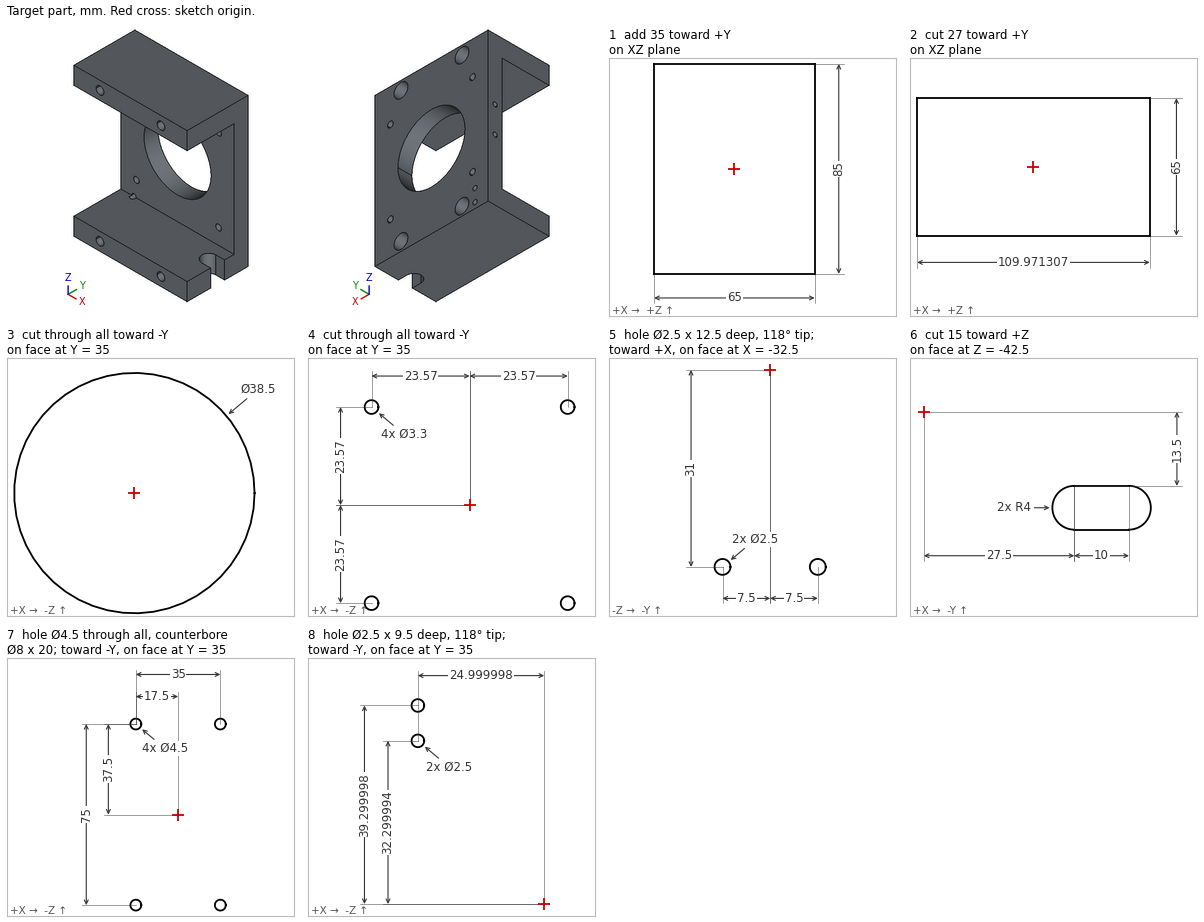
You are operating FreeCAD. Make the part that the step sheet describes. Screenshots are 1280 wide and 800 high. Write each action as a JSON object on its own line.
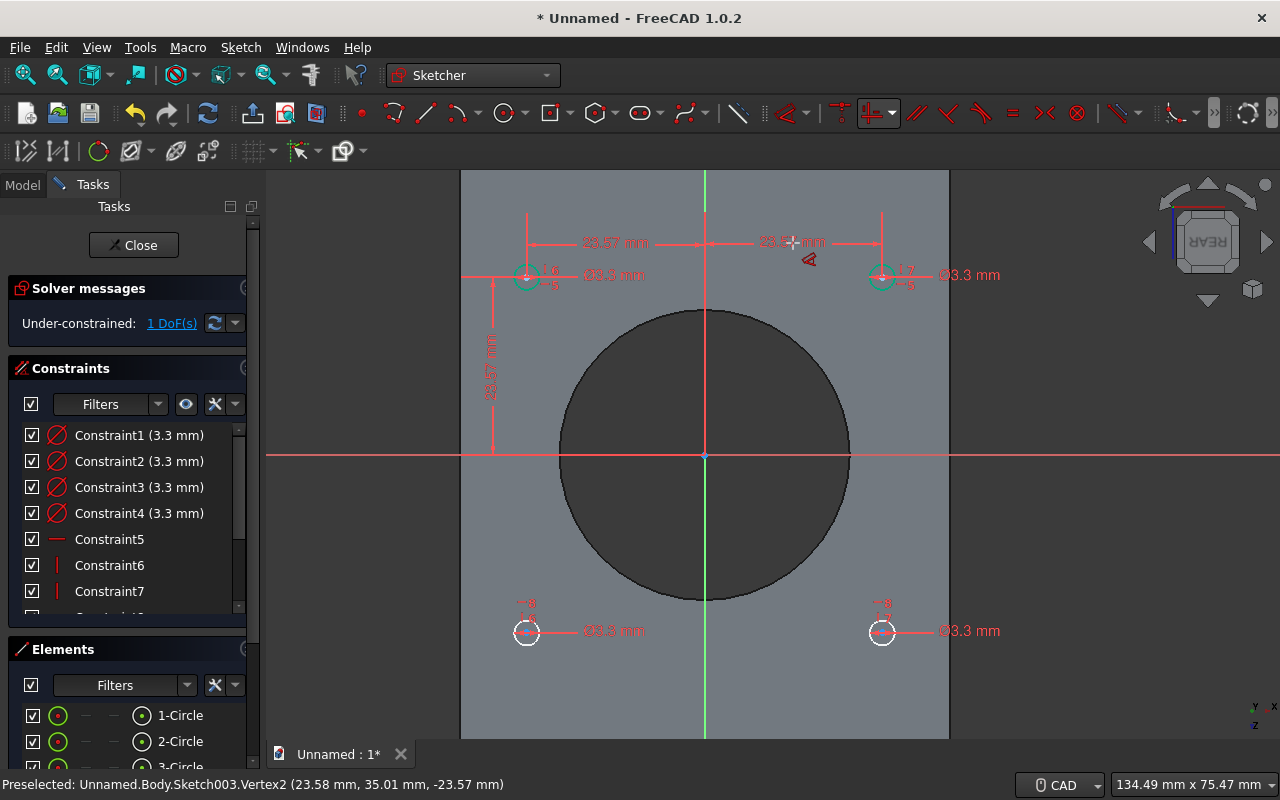
{"action": "left_click", "coordinate": [527, 633]}
{"action": "left_click", "coordinate": [493, 544]}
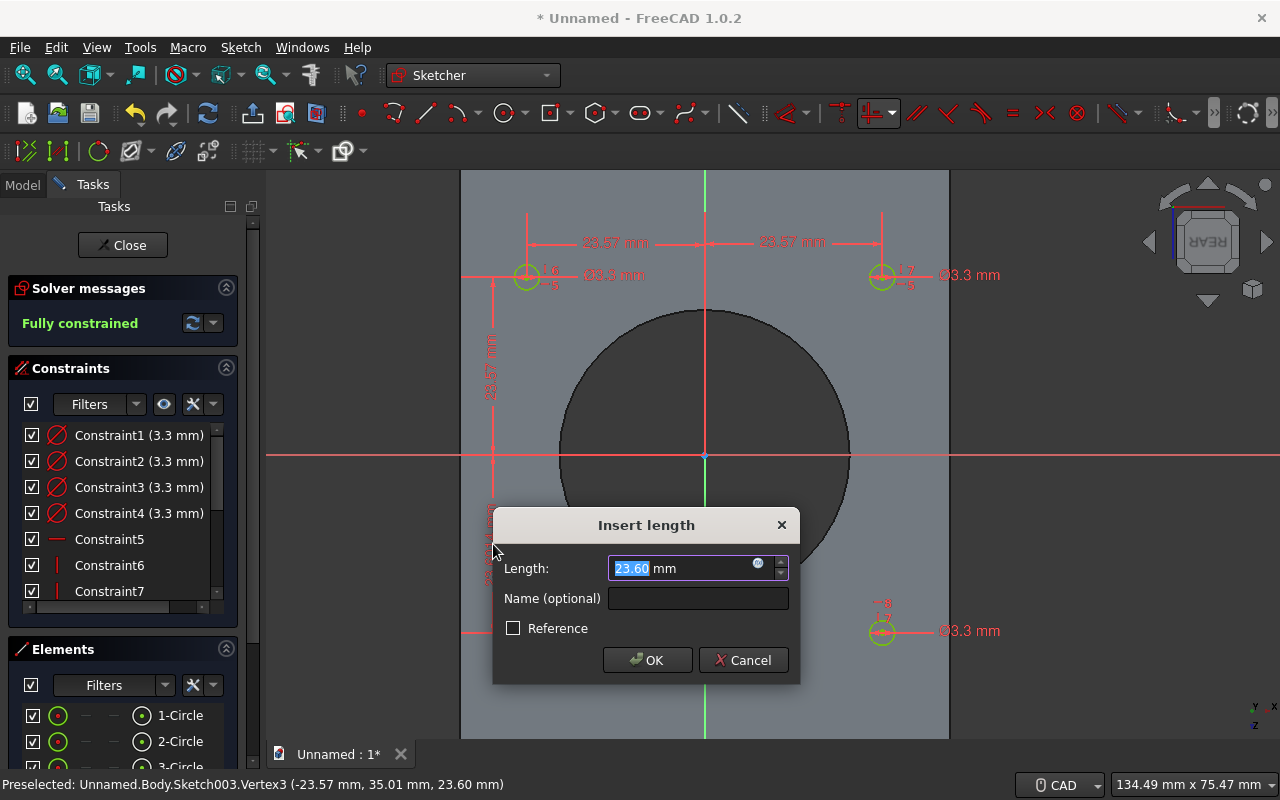
{"action": "type", "text": "23.57"}
{"action": "key", "text": "Return"}
{"action": "key", "text": "Escape"}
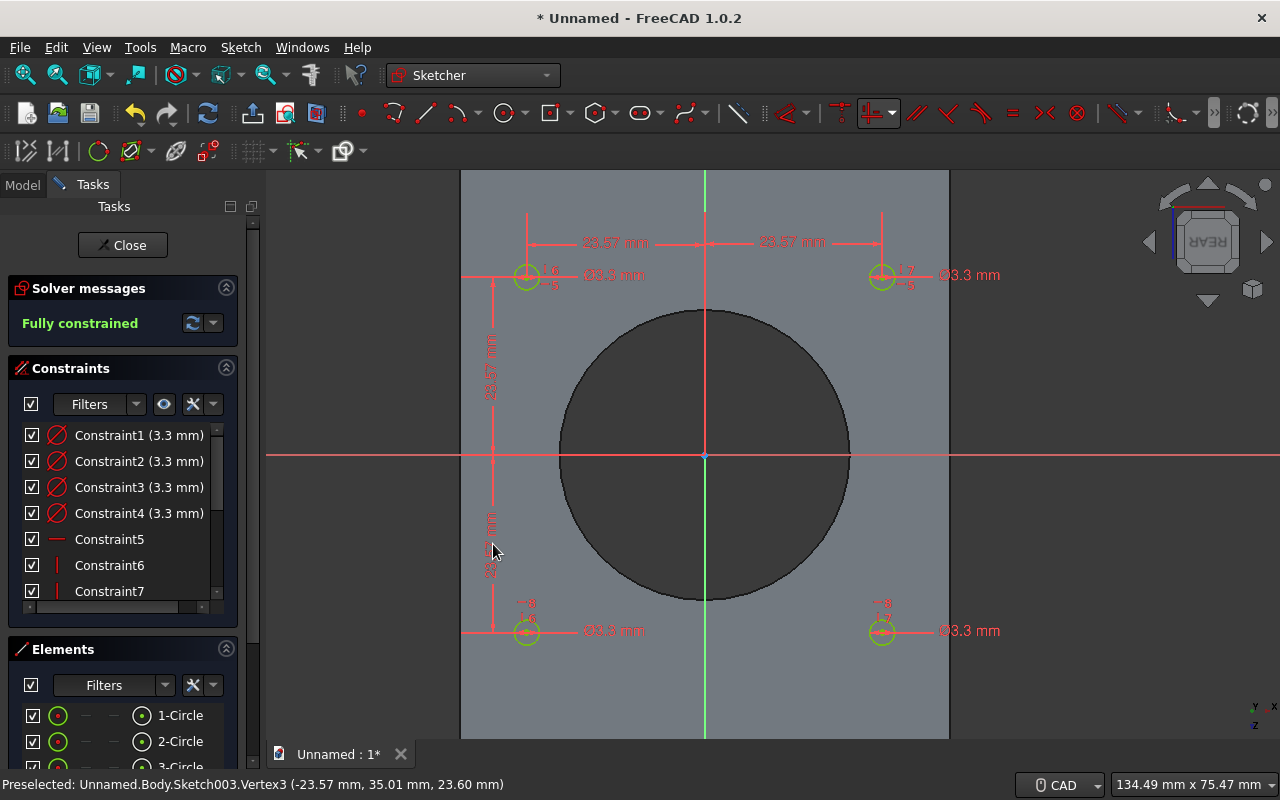
{"action": "left_click", "coordinate": [123, 245]}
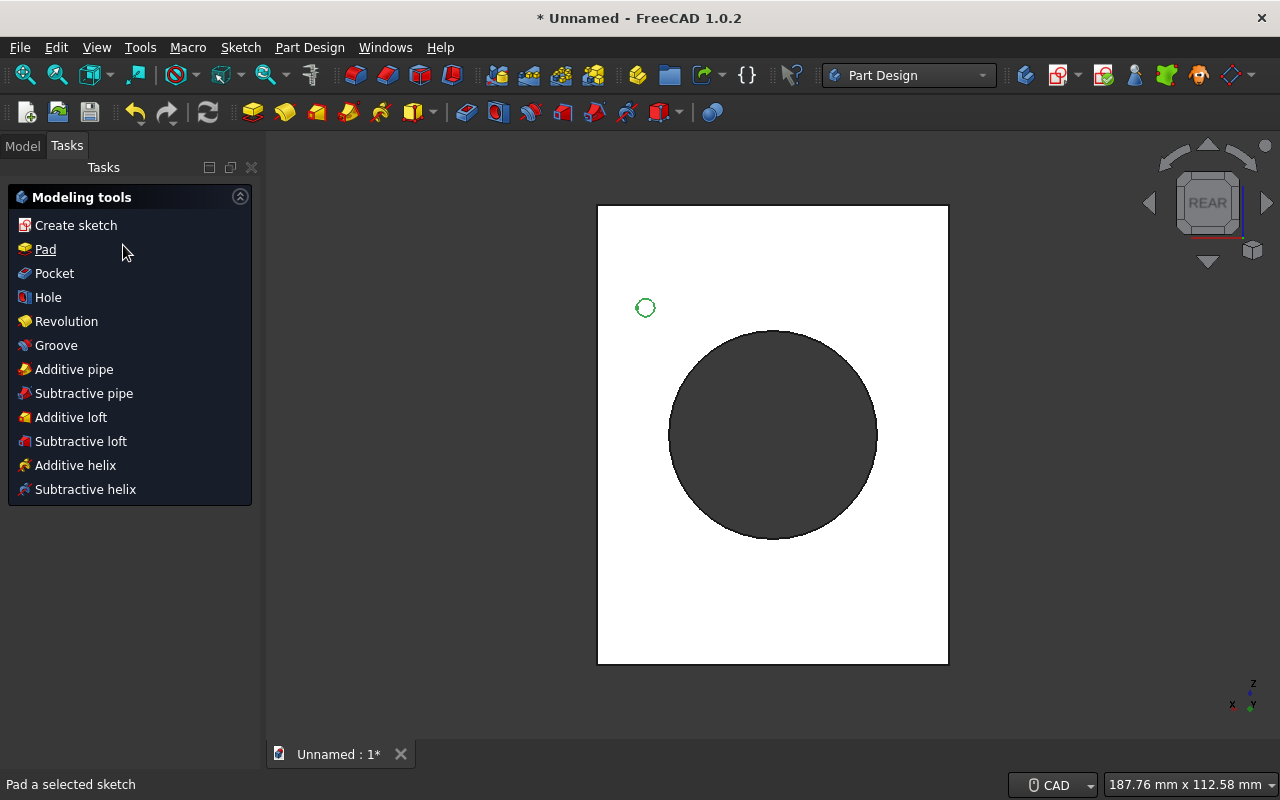
{"action": "left_click", "coordinate": [468, 112]}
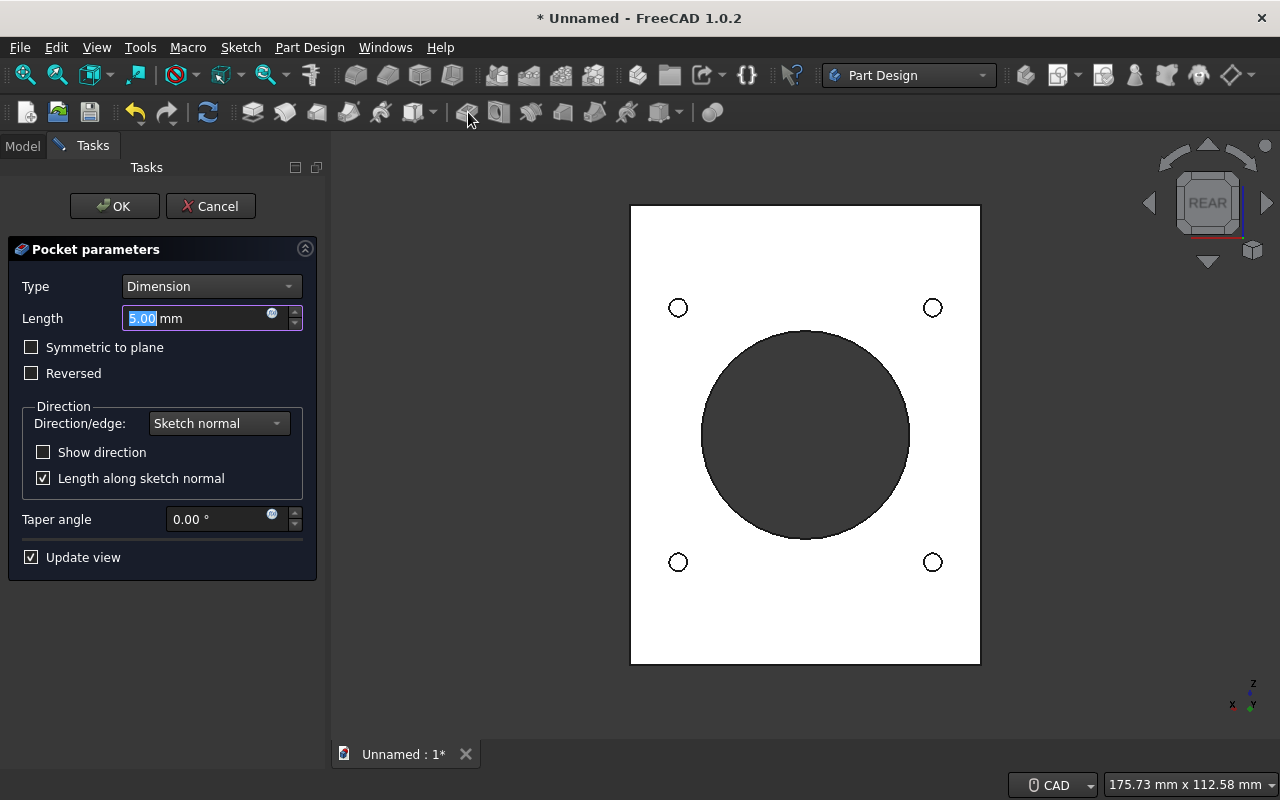
{"action": "left_click", "coordinate": [212, 286]}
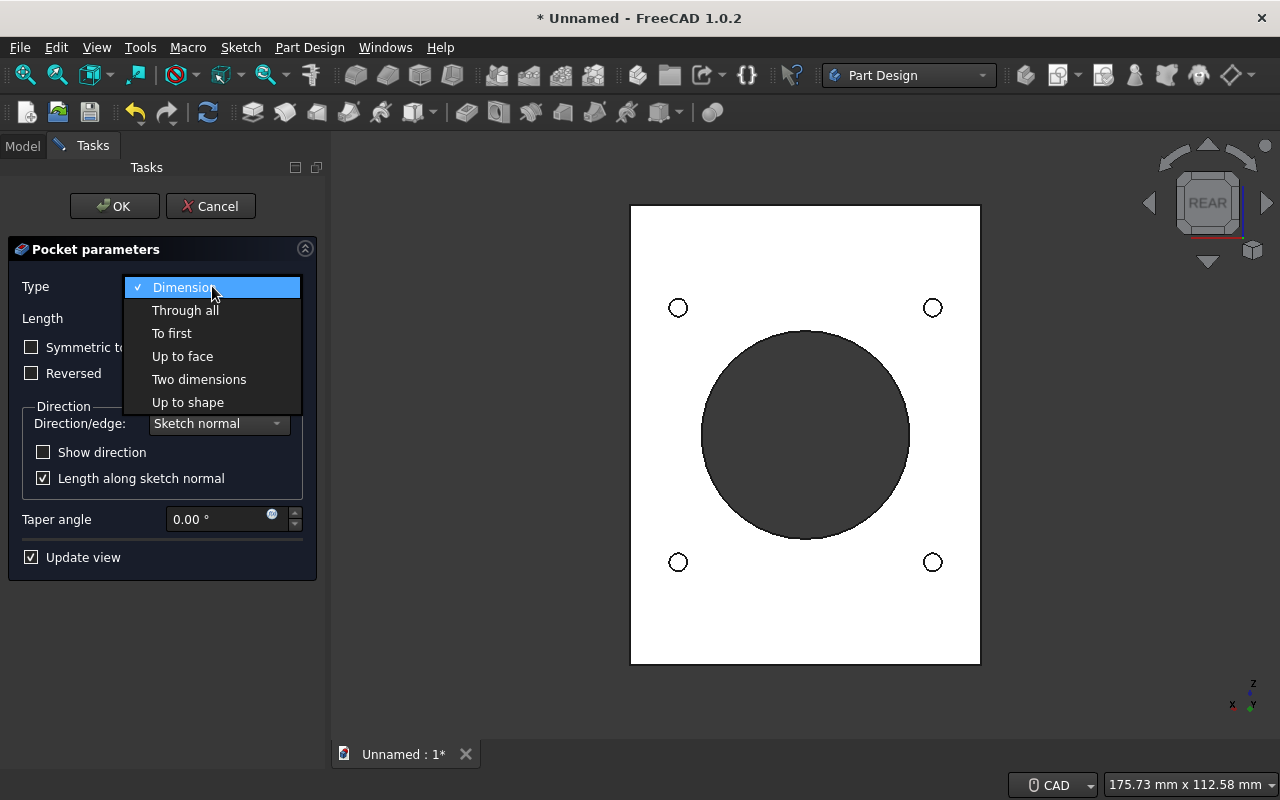
{"action": "left_click", "coordinate": [212, 310]}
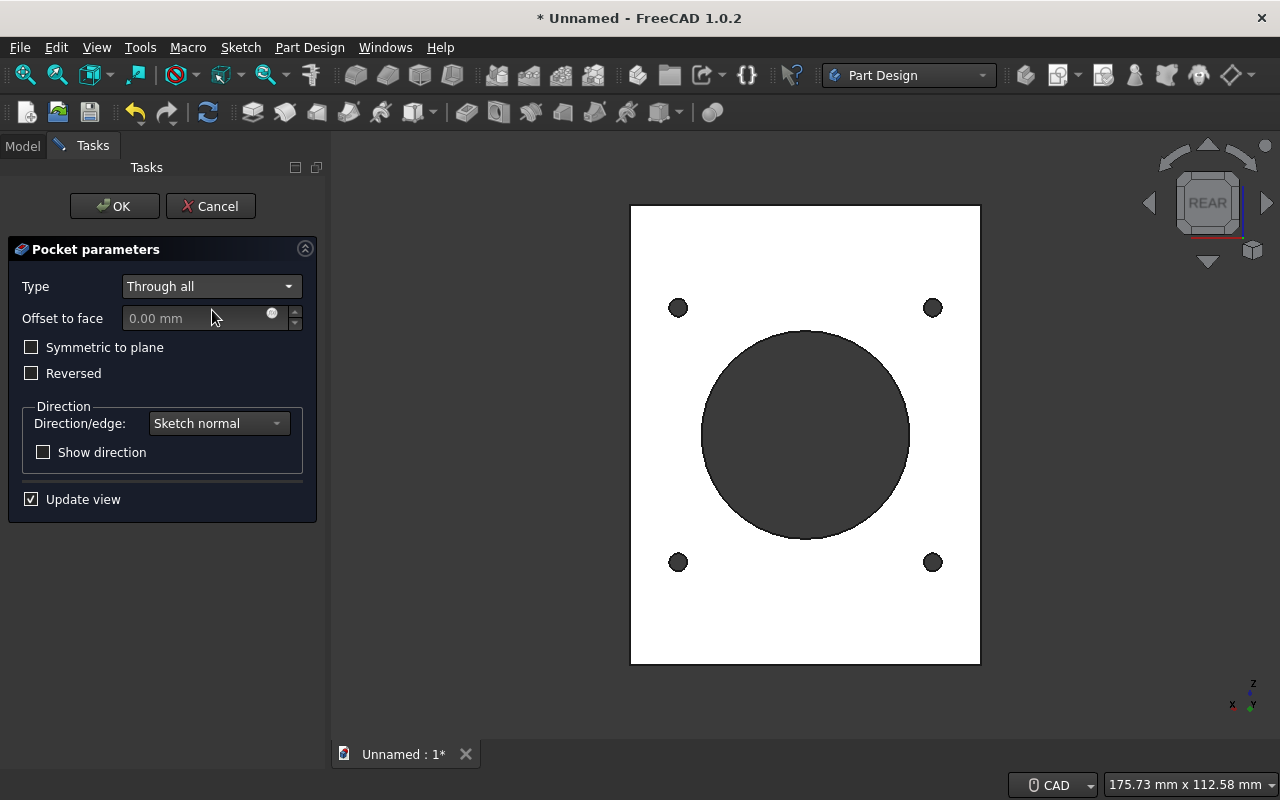
{"action": "left_click", "coordinate": [115, 206]}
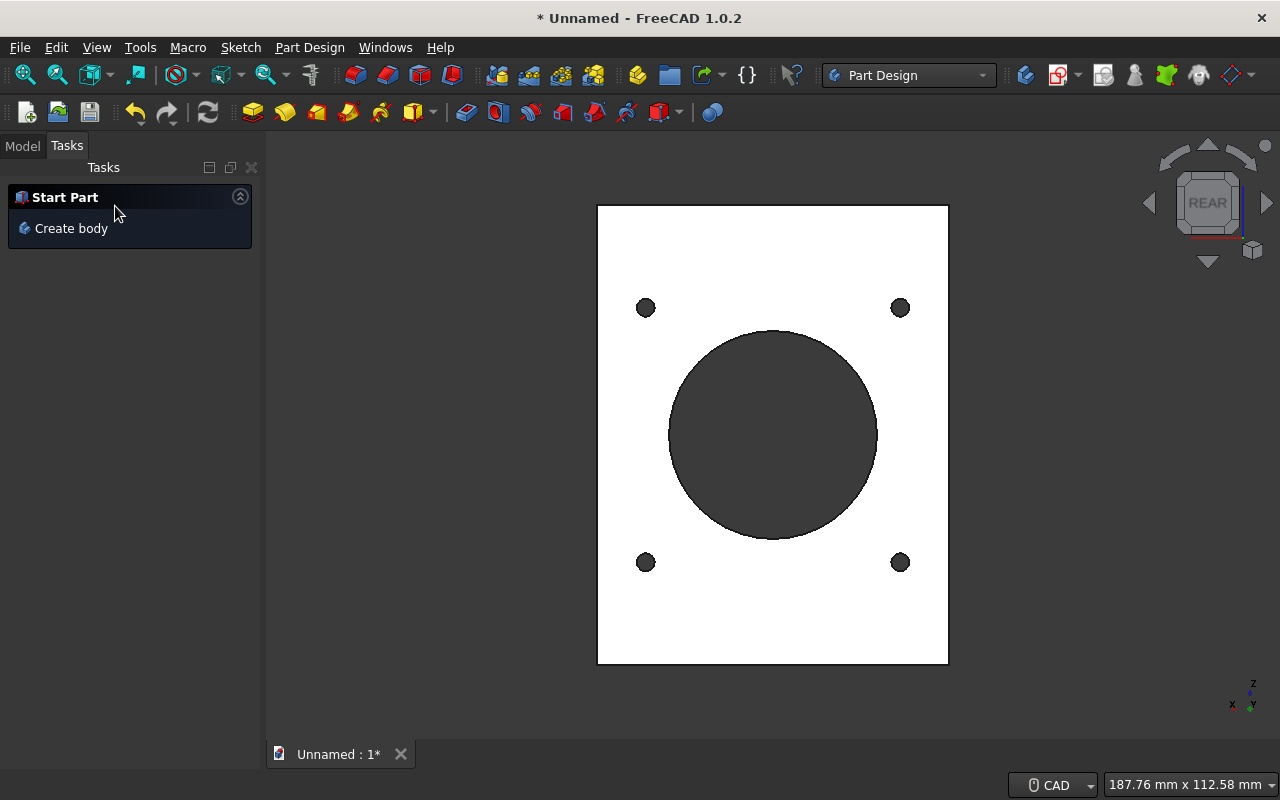
{"action": "key", "text": "6"}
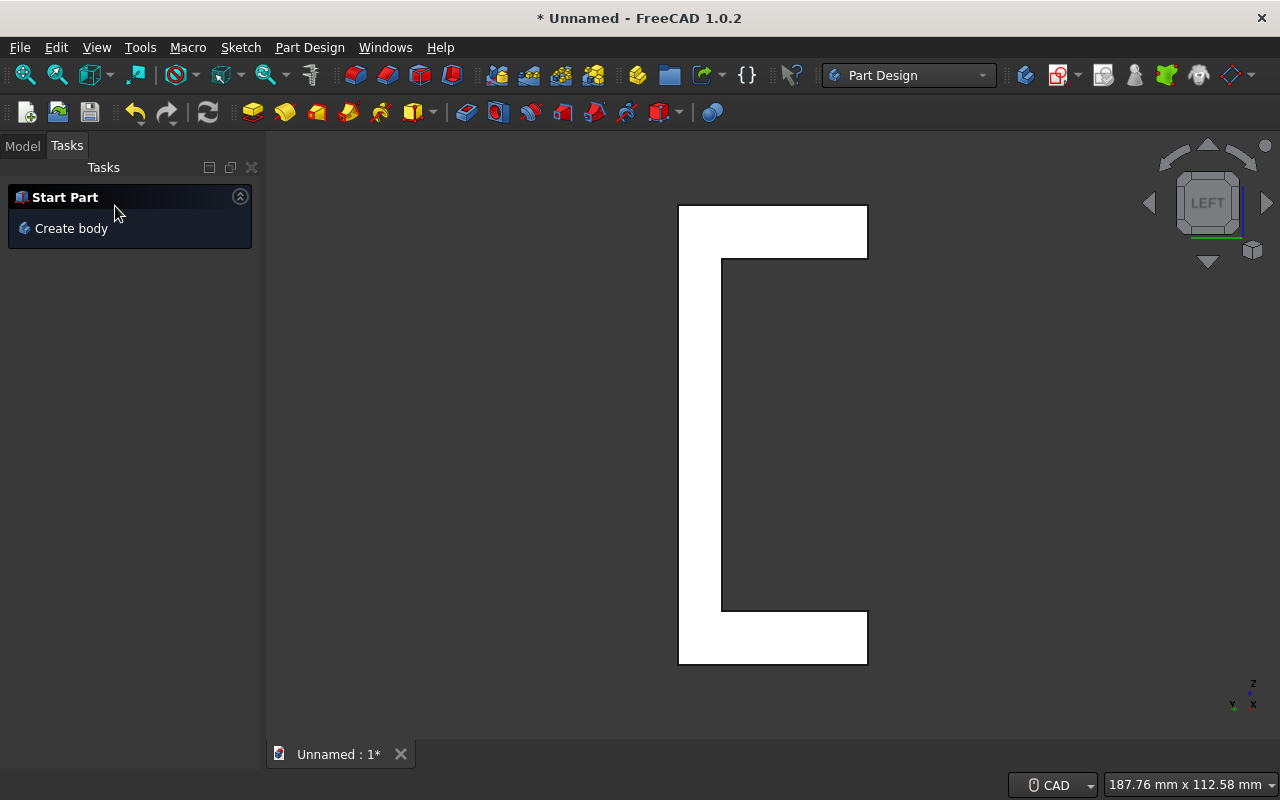
{"action": "left_click", "coordinate": [719, 237]}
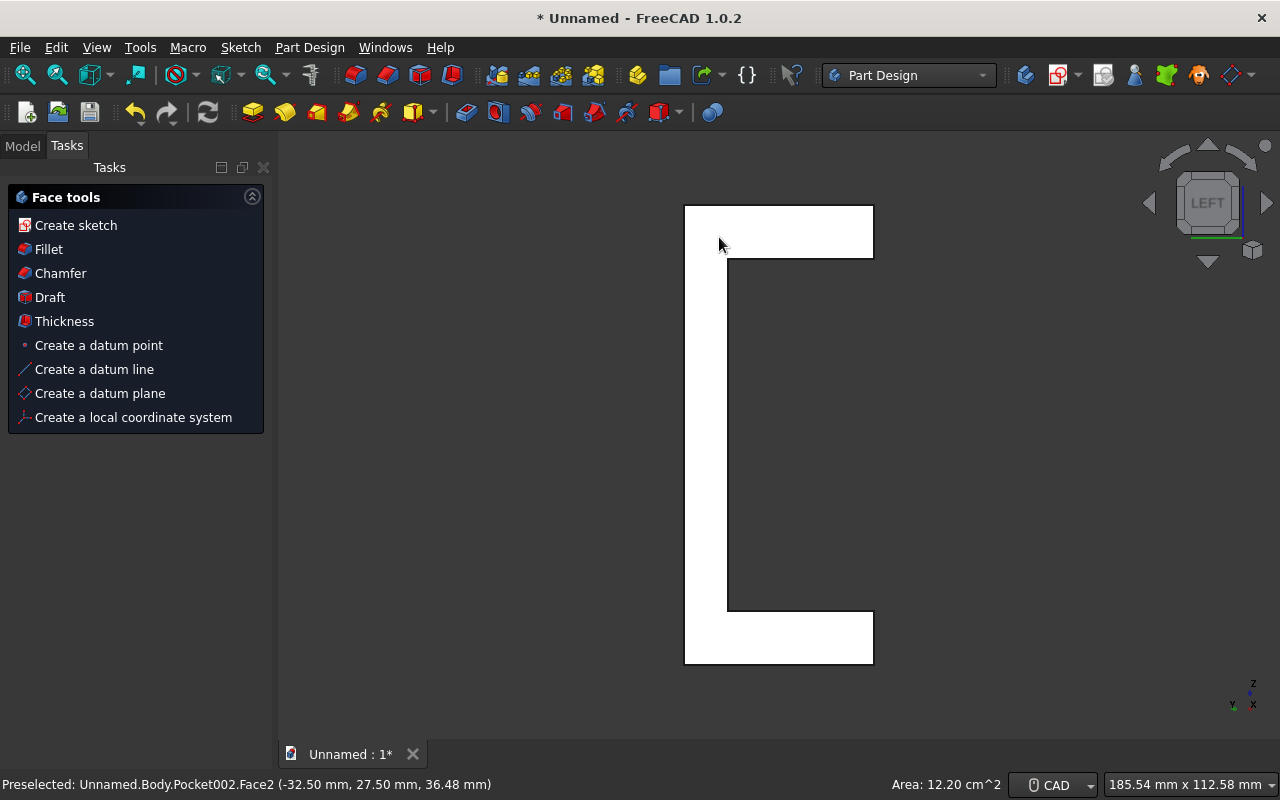
{"action": "left_click", "coordinate": [1058, 76]}